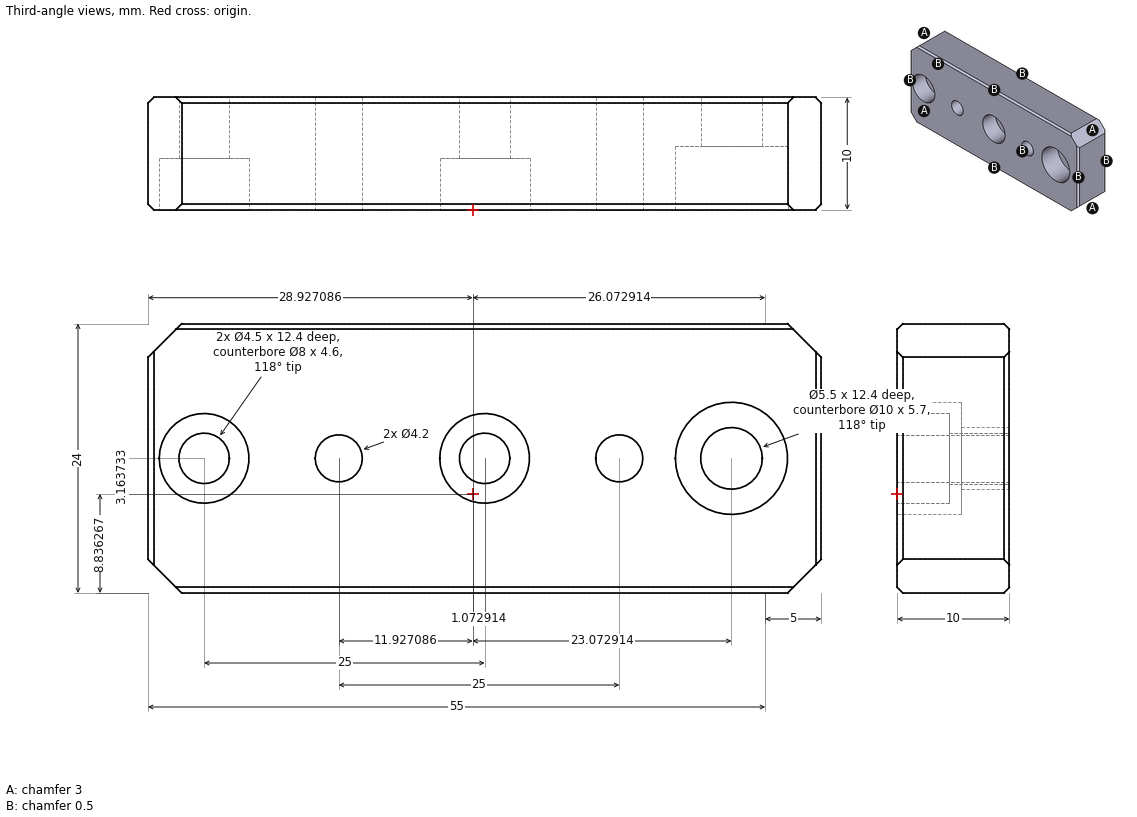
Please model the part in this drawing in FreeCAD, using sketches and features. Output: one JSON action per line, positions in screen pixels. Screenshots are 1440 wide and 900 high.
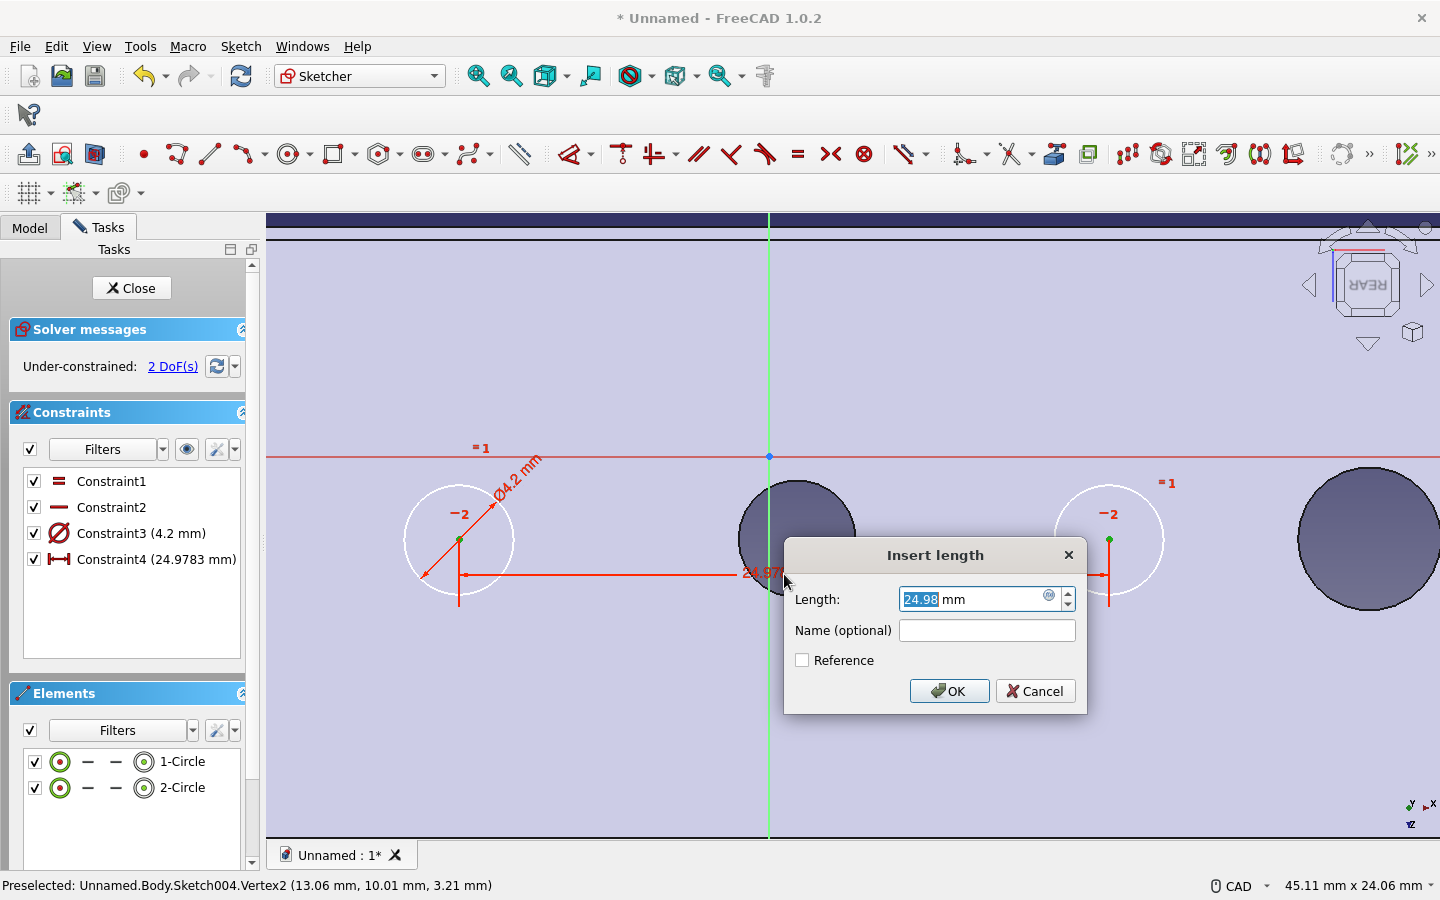
{"action": "type", "text": "25"}
{"action": "key", "text": "Return"}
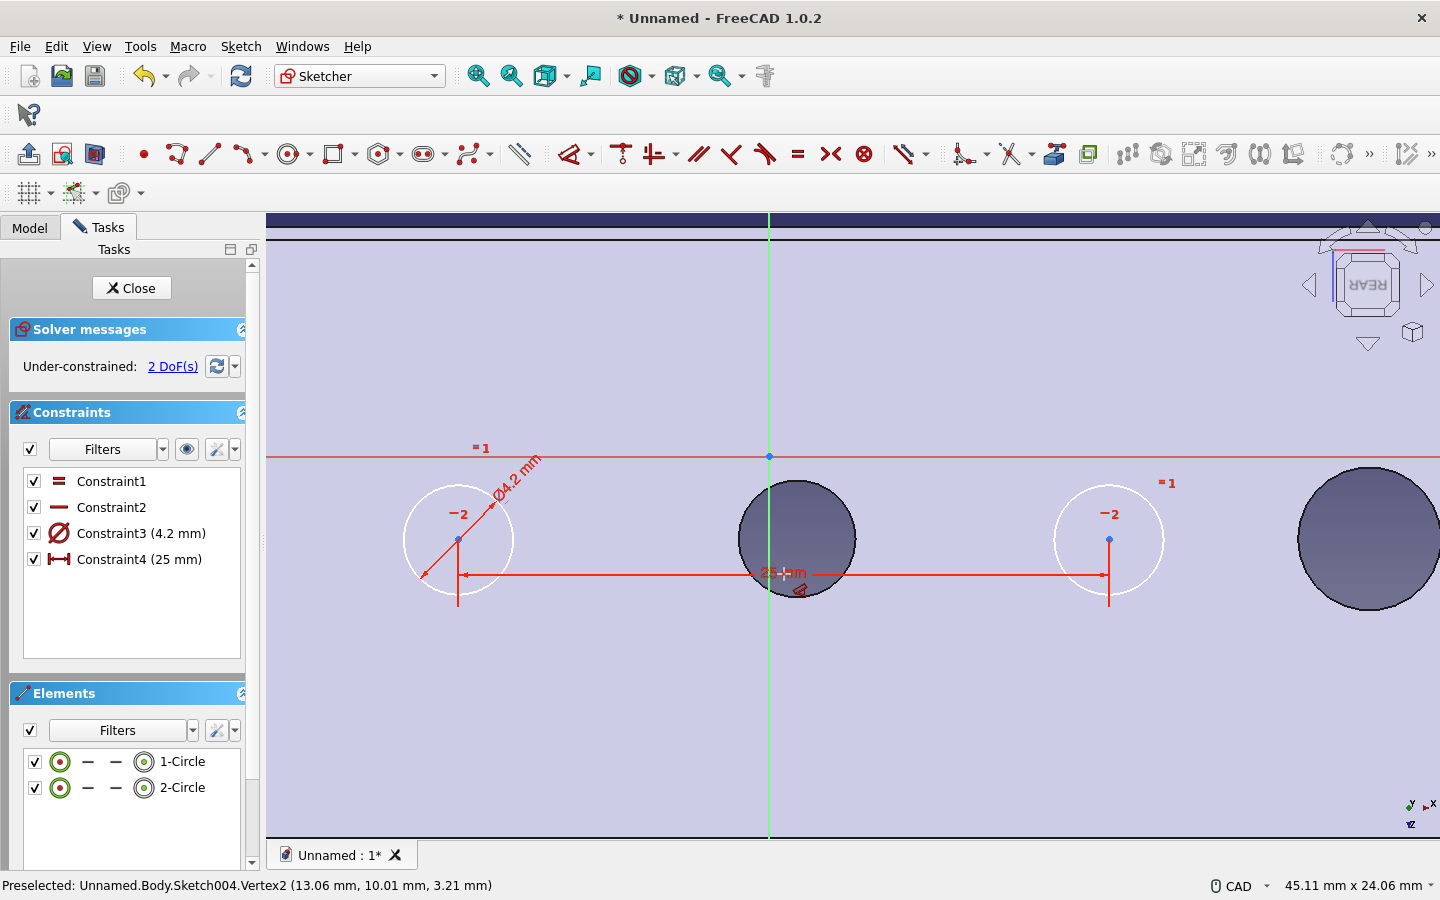
{"action": "left_click", "coordinate": [458, 540]}
{"action": "left_click", "coordinate": [424, 479]}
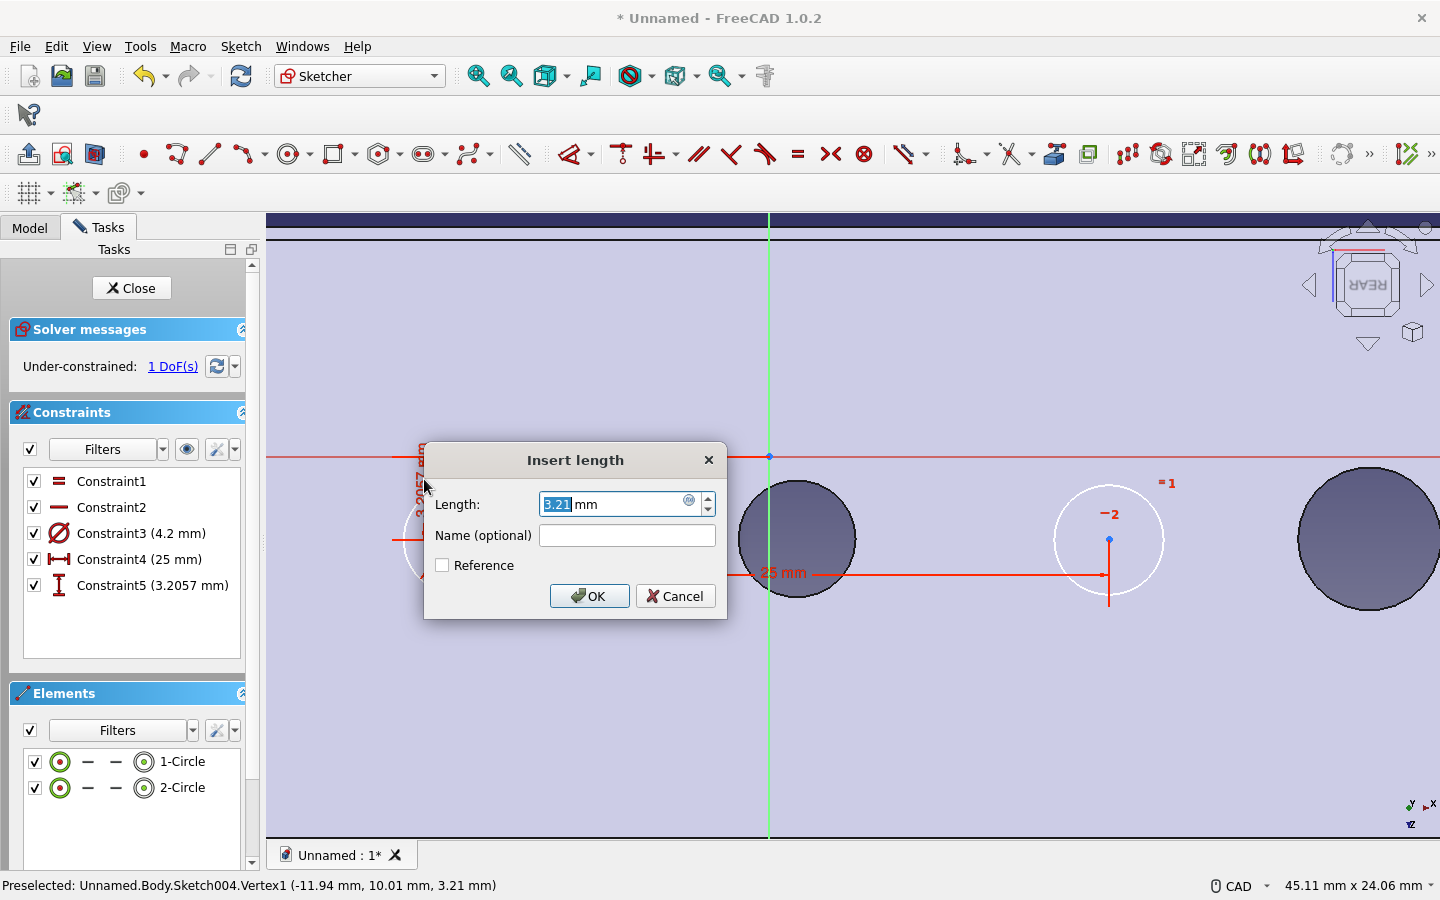
{"action": "type", "text": "3.163733"}
{"action": "key", "text": "Return"}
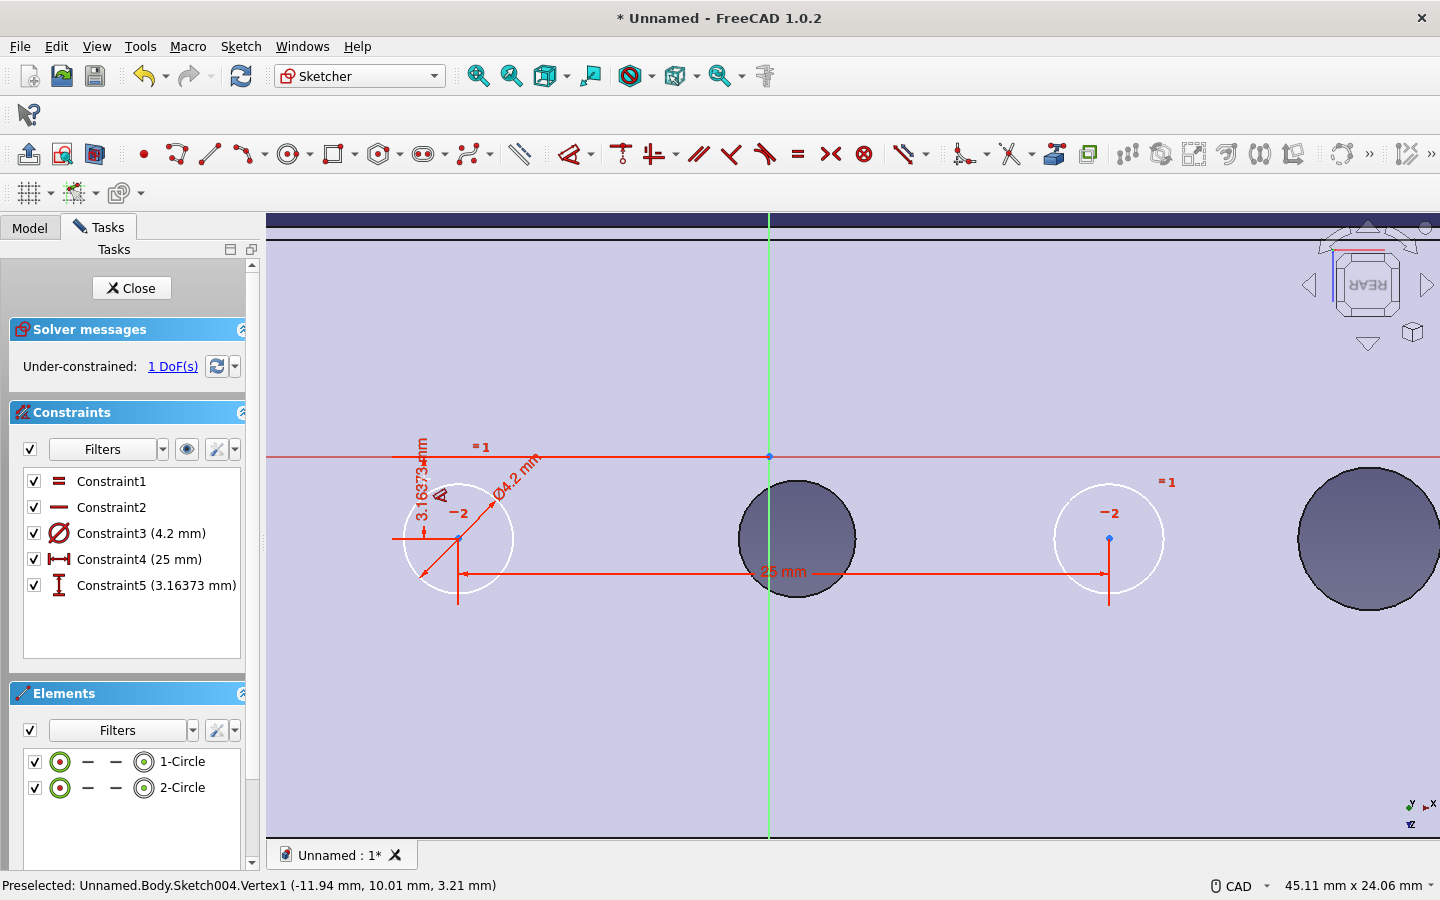
{"action": "left_click", "coordinate": [458, 539]}
{"action": "left_click", "coordinate": [614, 423]}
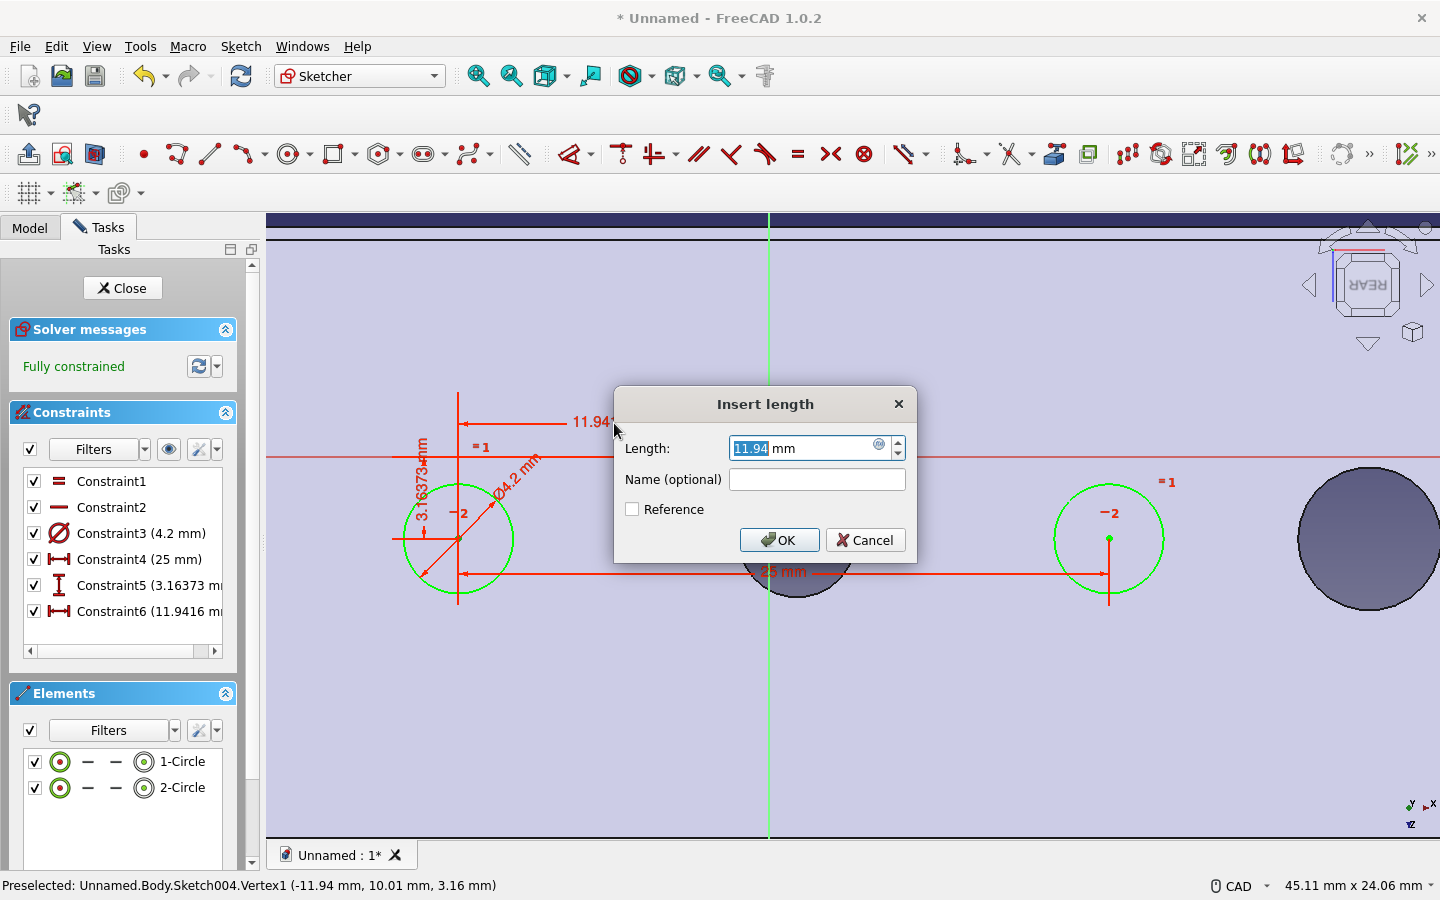
{"action": "type", "text": "11.927086"}
{"action": "key", "text": "Return"}
{"action": "key", "text": "Escape"}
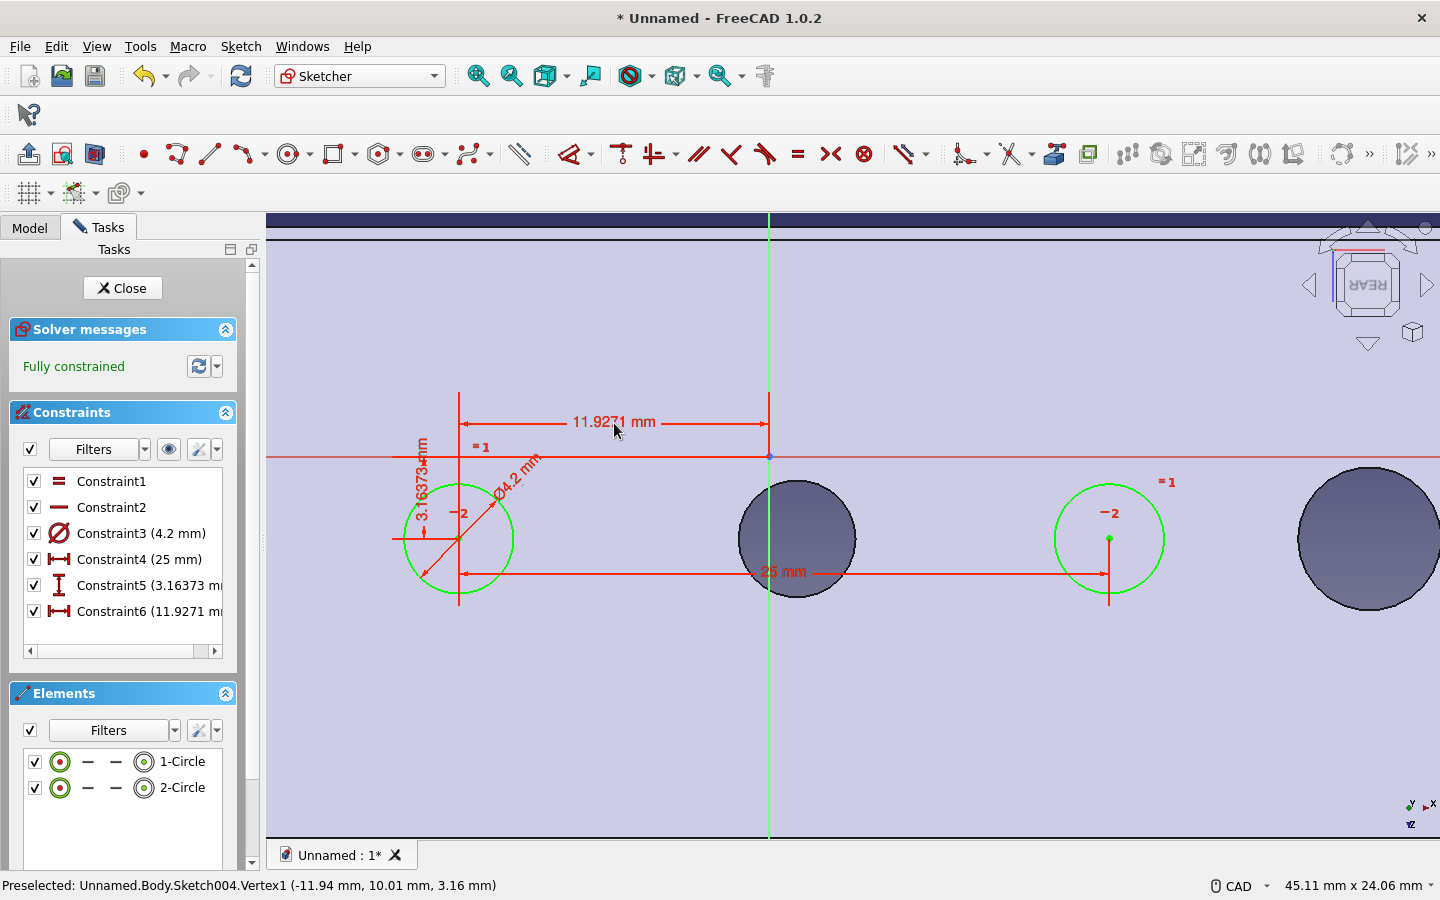
{"action": "left_click", "coordinate": [123, 288]}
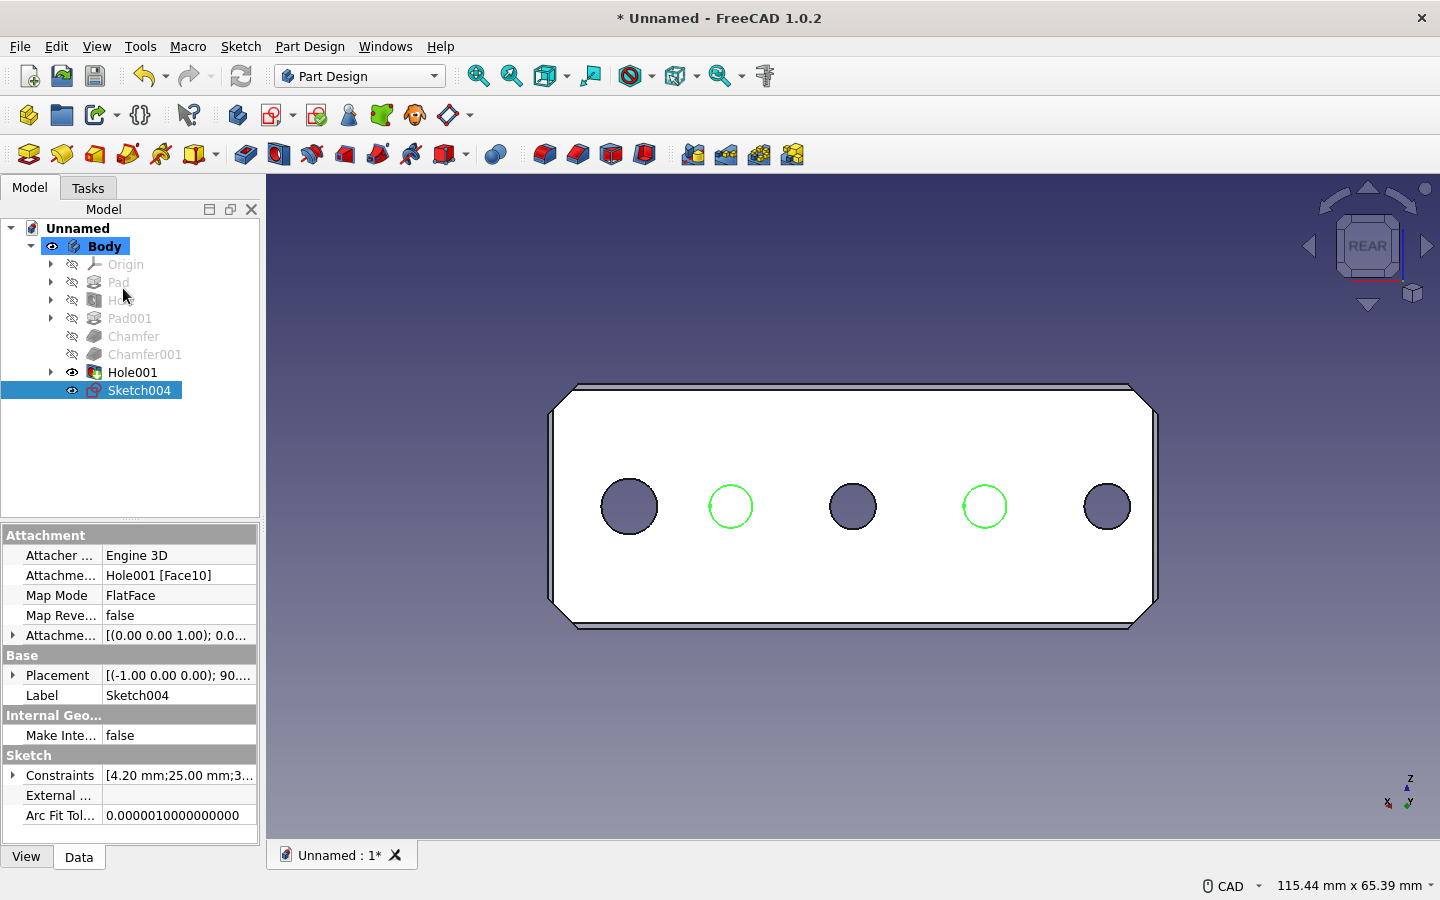
{"action": "left_click", "coordinate": [246, 154]}